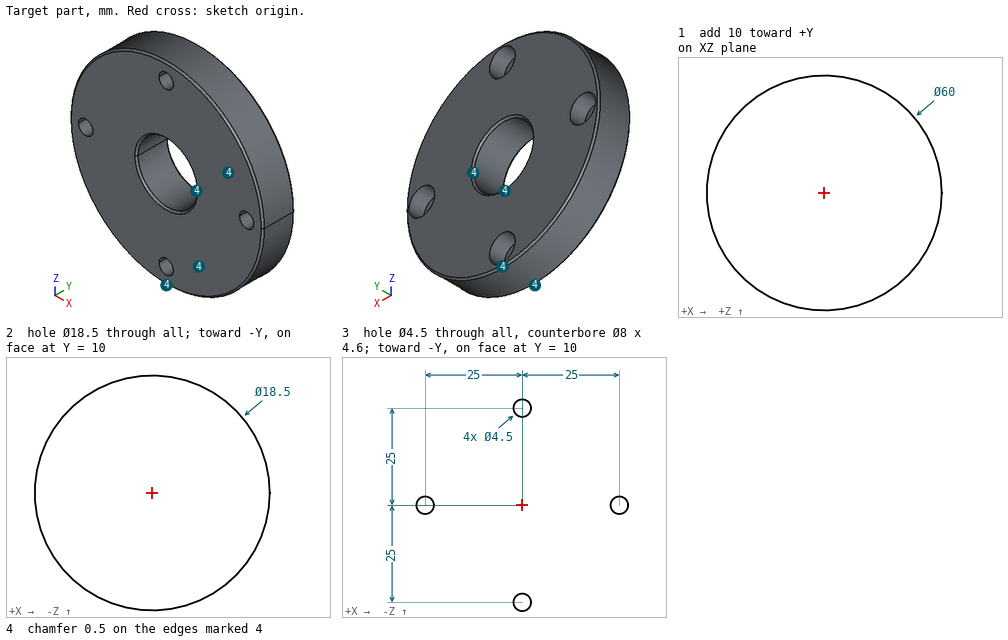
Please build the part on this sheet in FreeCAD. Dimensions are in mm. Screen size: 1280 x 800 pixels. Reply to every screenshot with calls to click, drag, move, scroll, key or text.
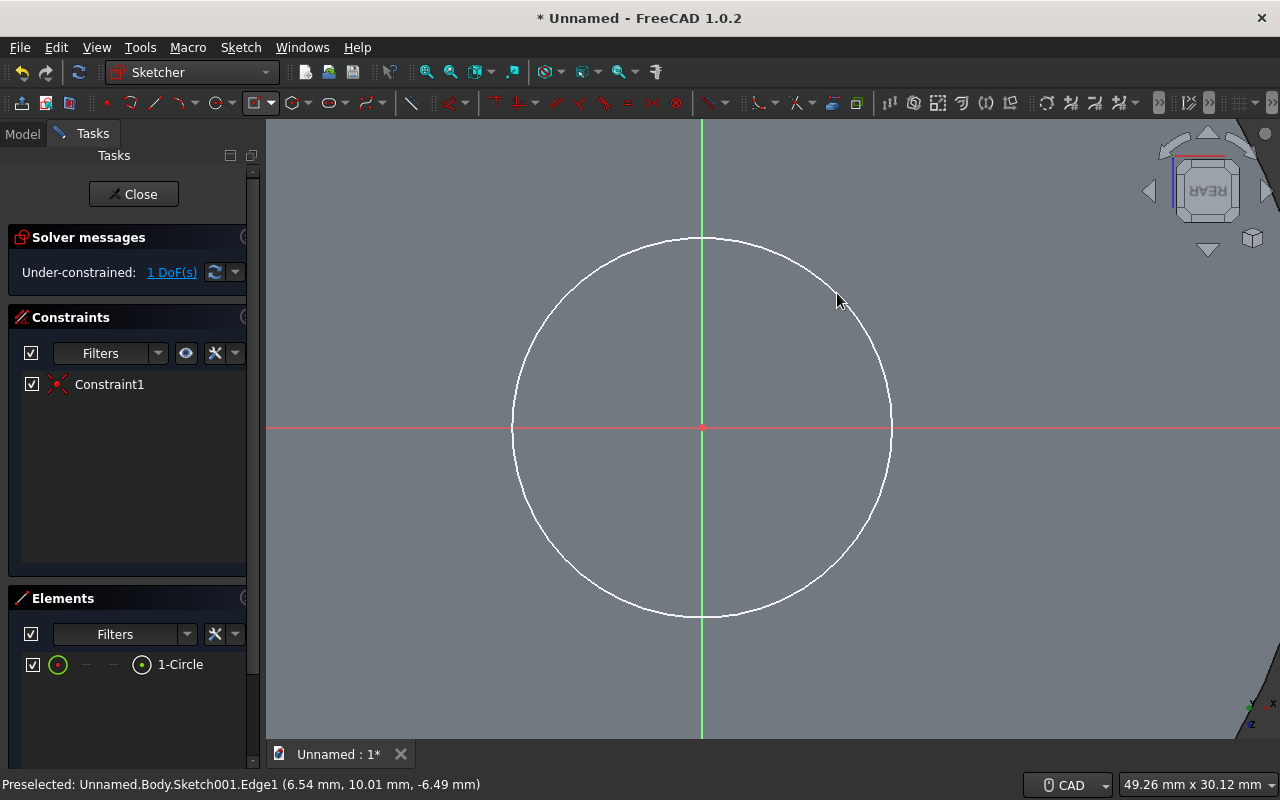
key(d)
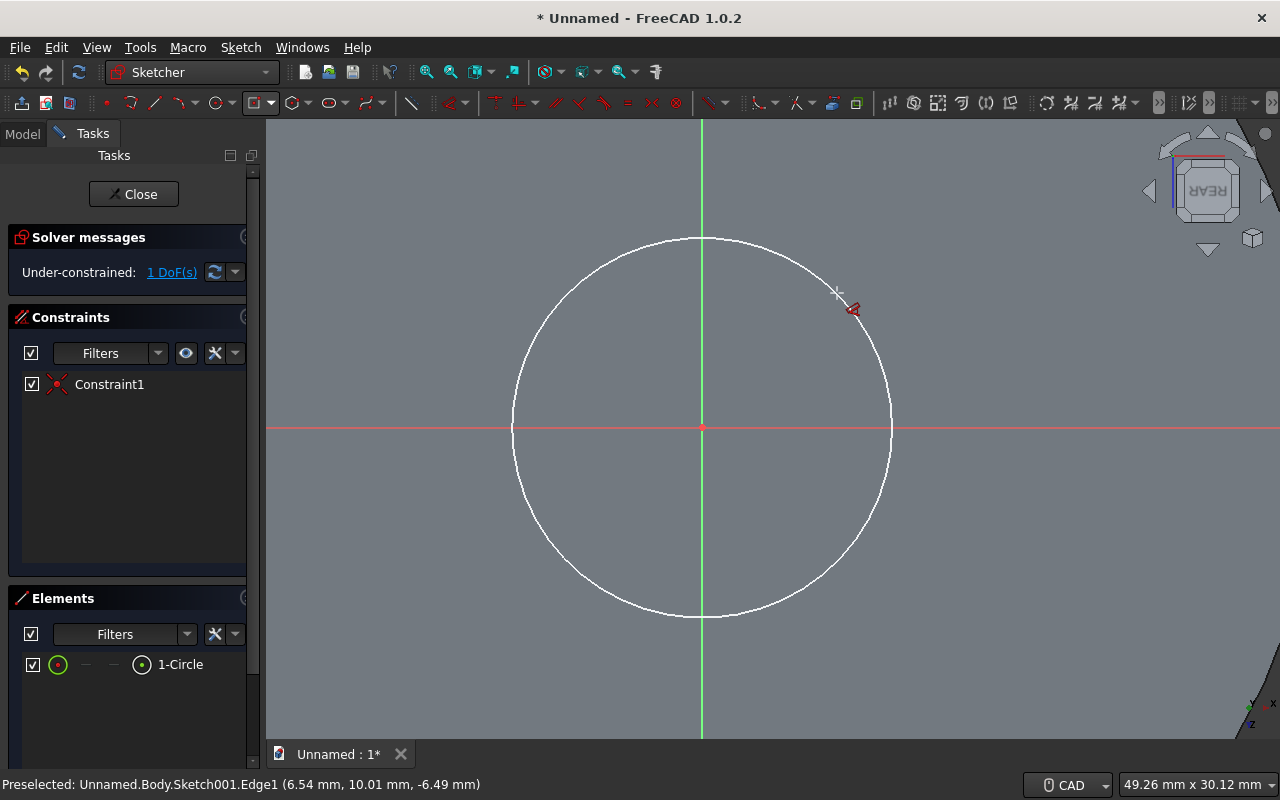
click(836, 293)
click(859, 270)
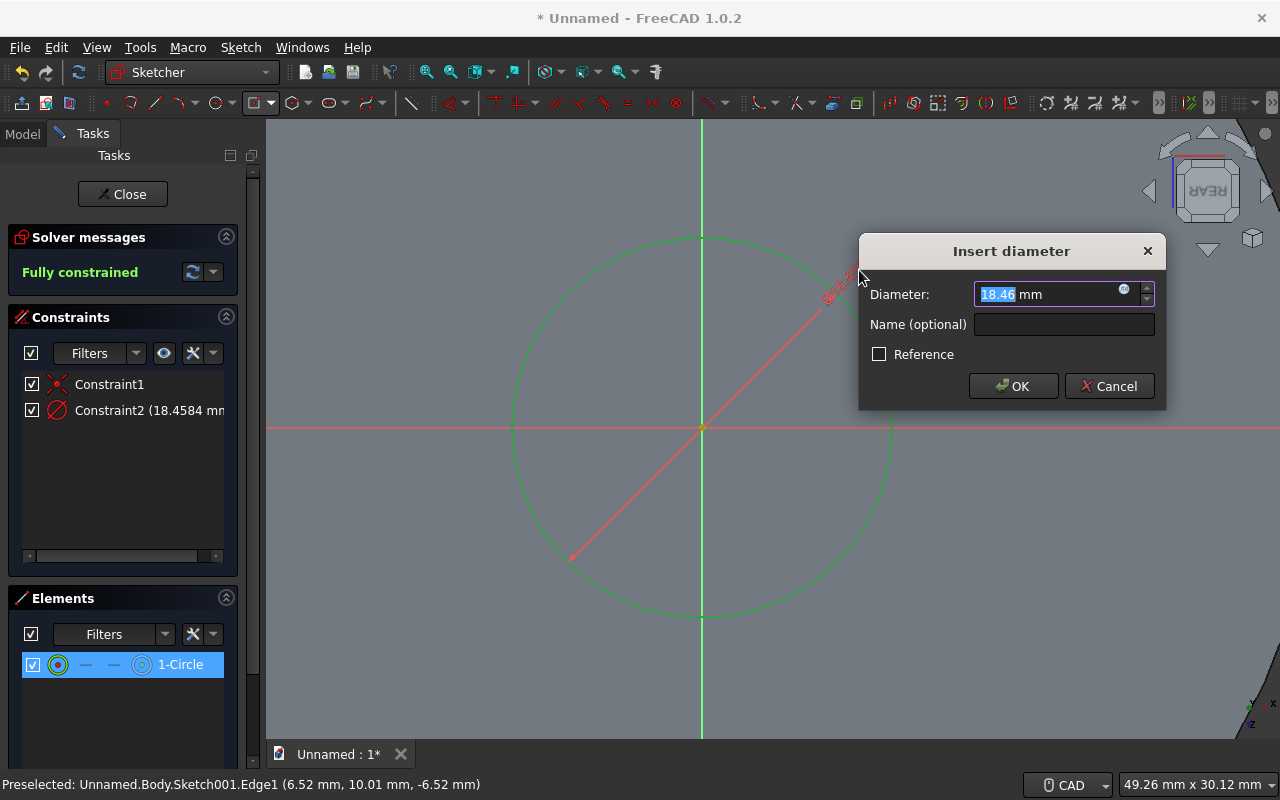
text(18.5)
key(Return)
key(Escape)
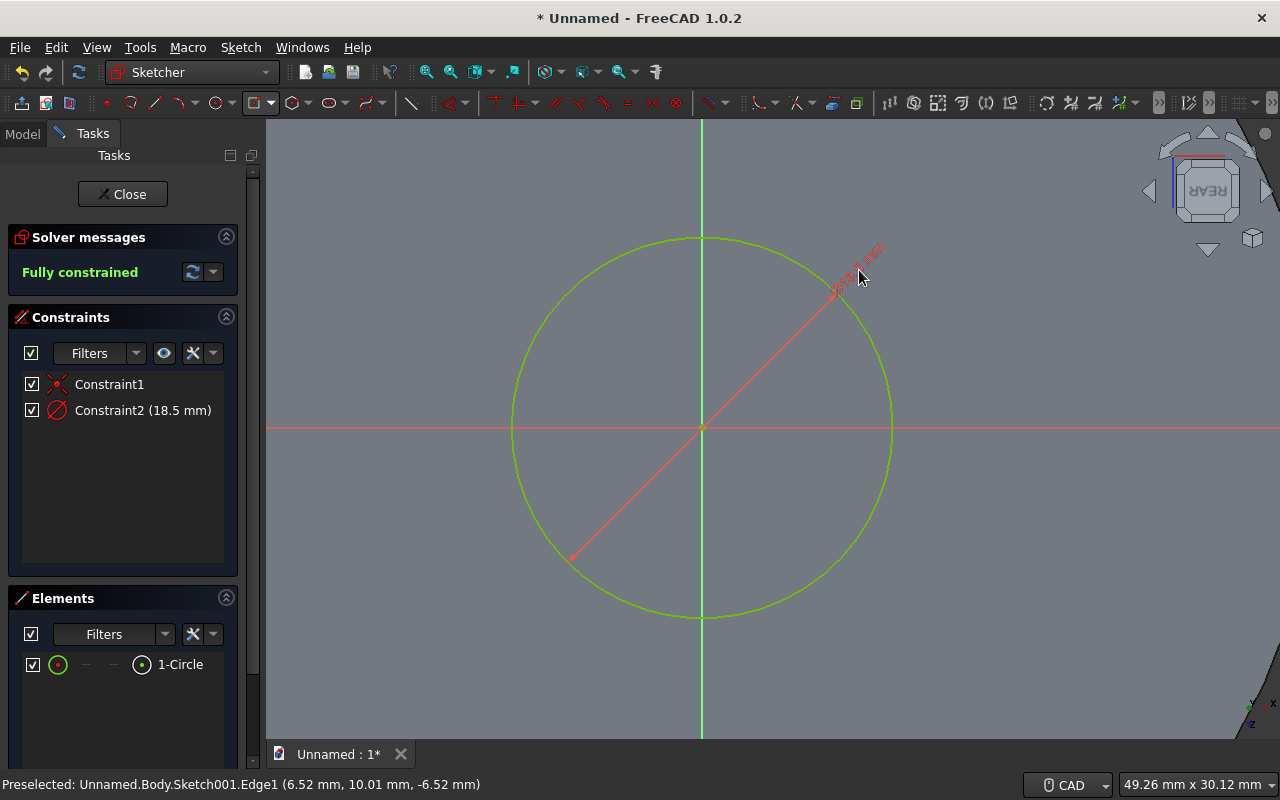
click(123, 194)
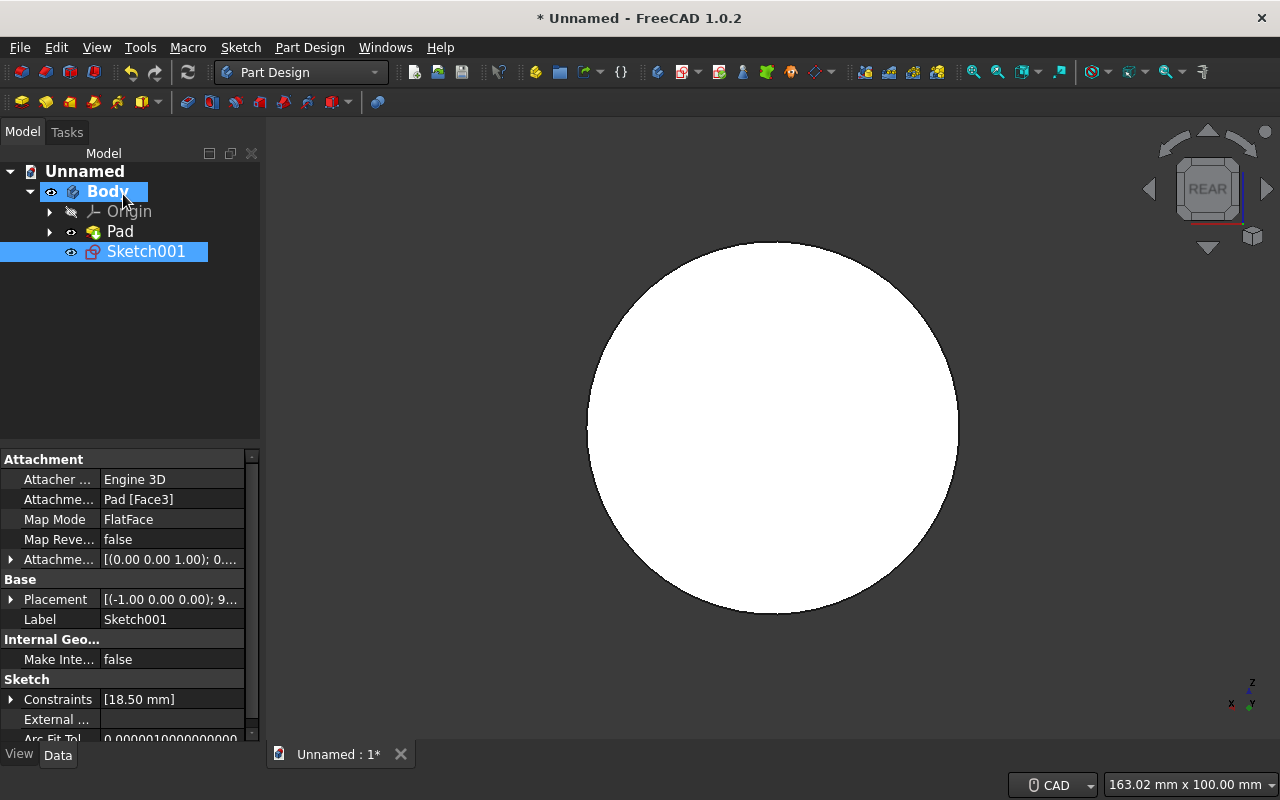
click(212, 102)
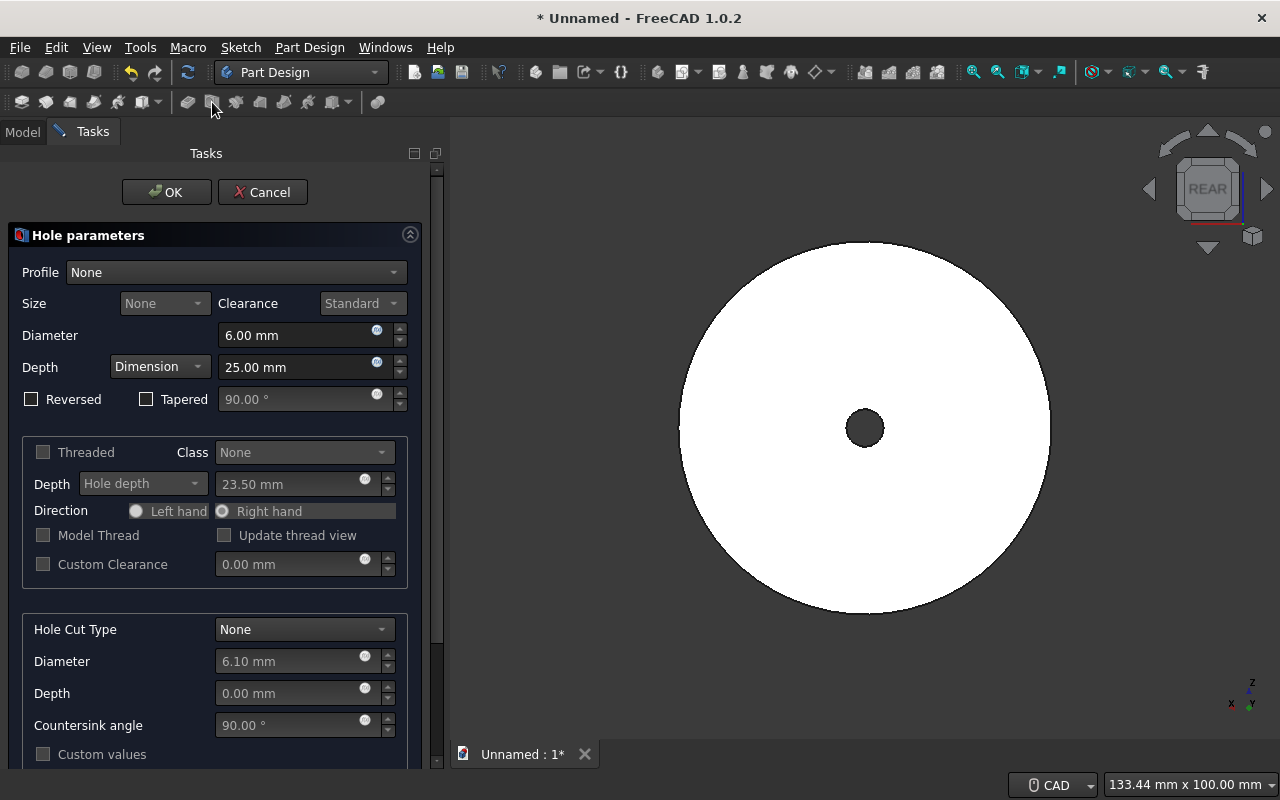
triple_click(305, 335)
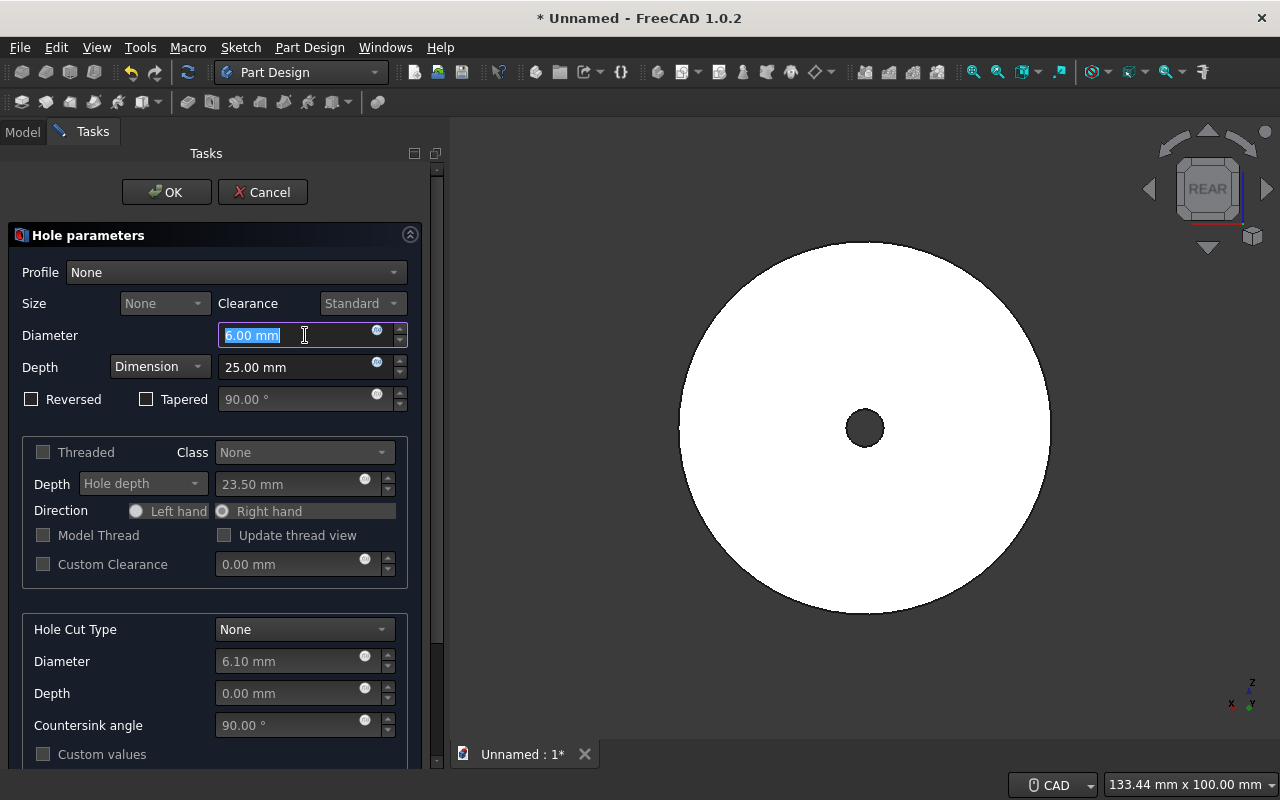
text(18.5)
key(Tab)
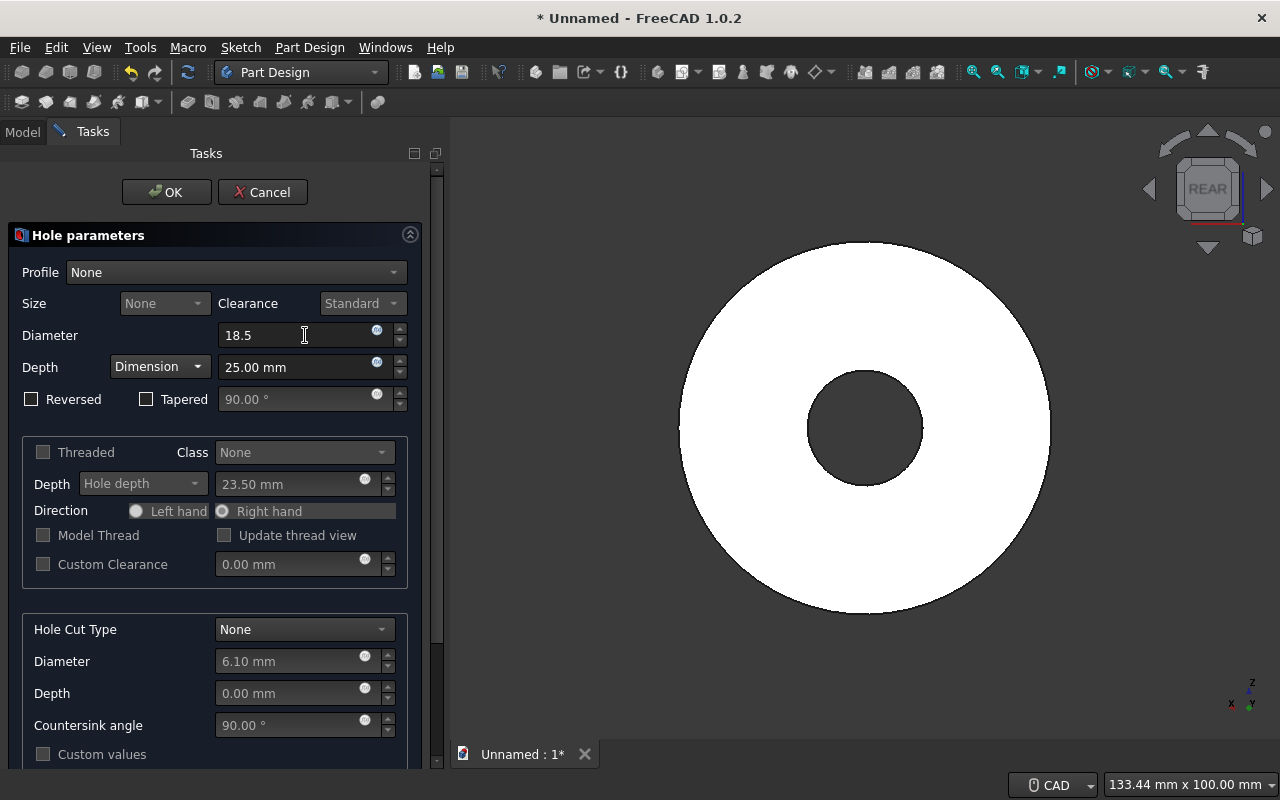
click(161, 366)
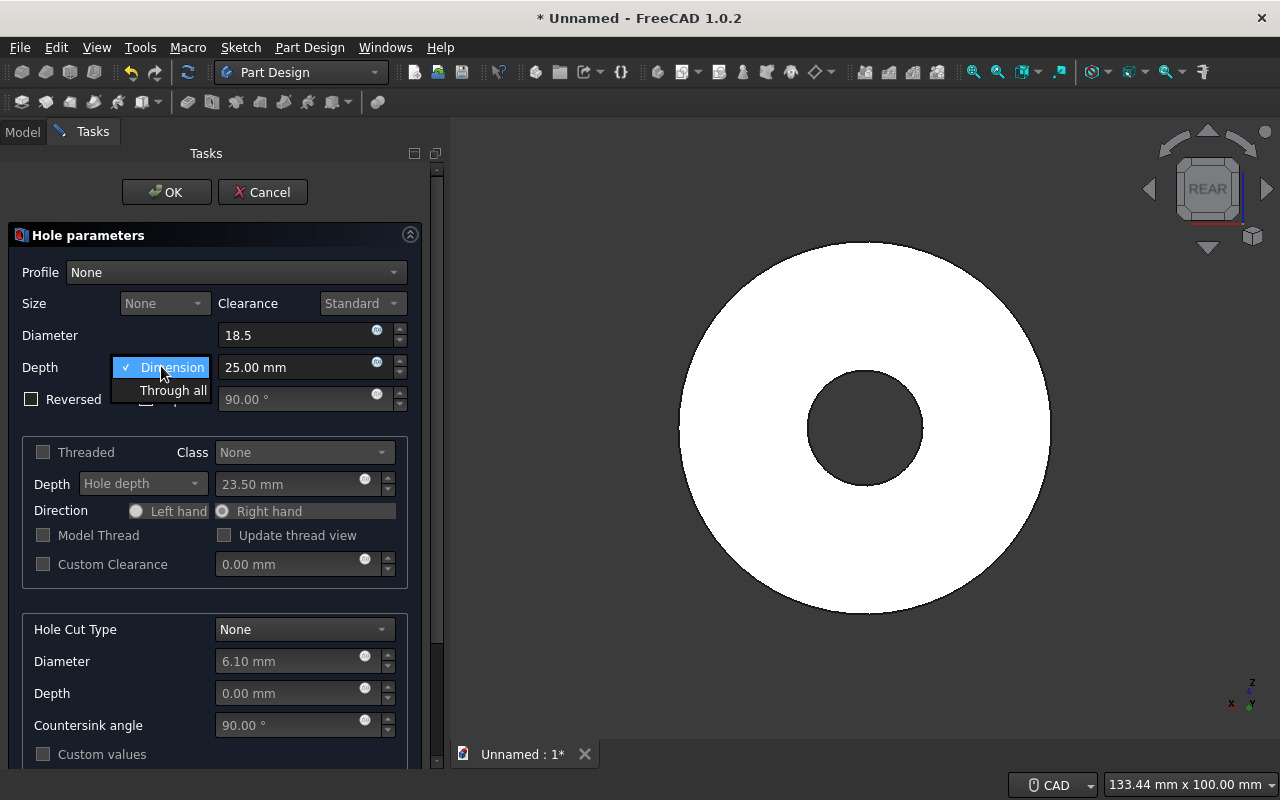
click(160, 390)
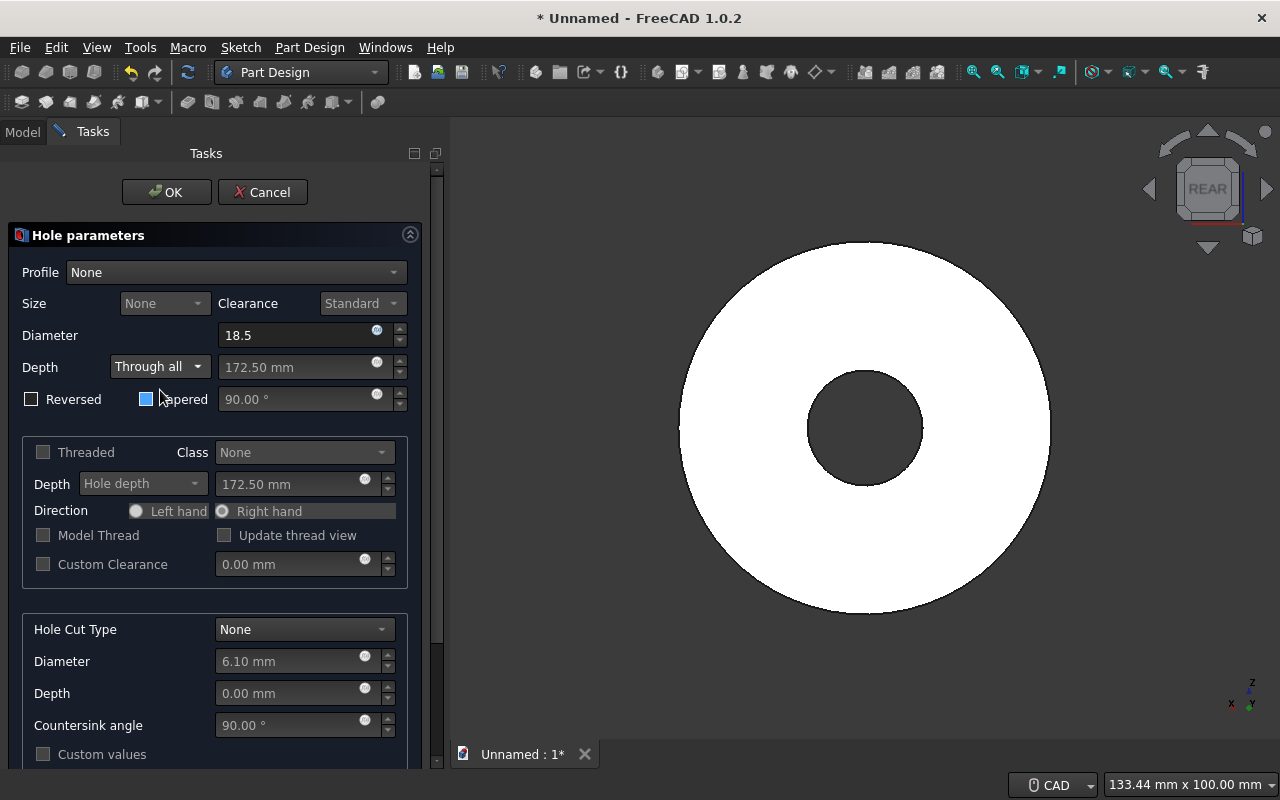
click(167, 192)